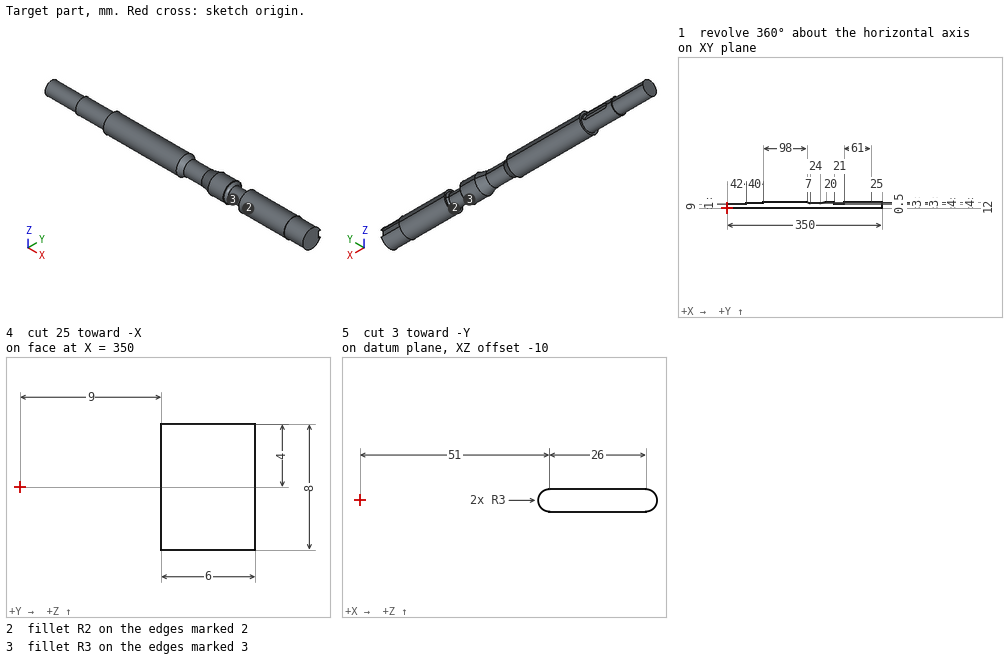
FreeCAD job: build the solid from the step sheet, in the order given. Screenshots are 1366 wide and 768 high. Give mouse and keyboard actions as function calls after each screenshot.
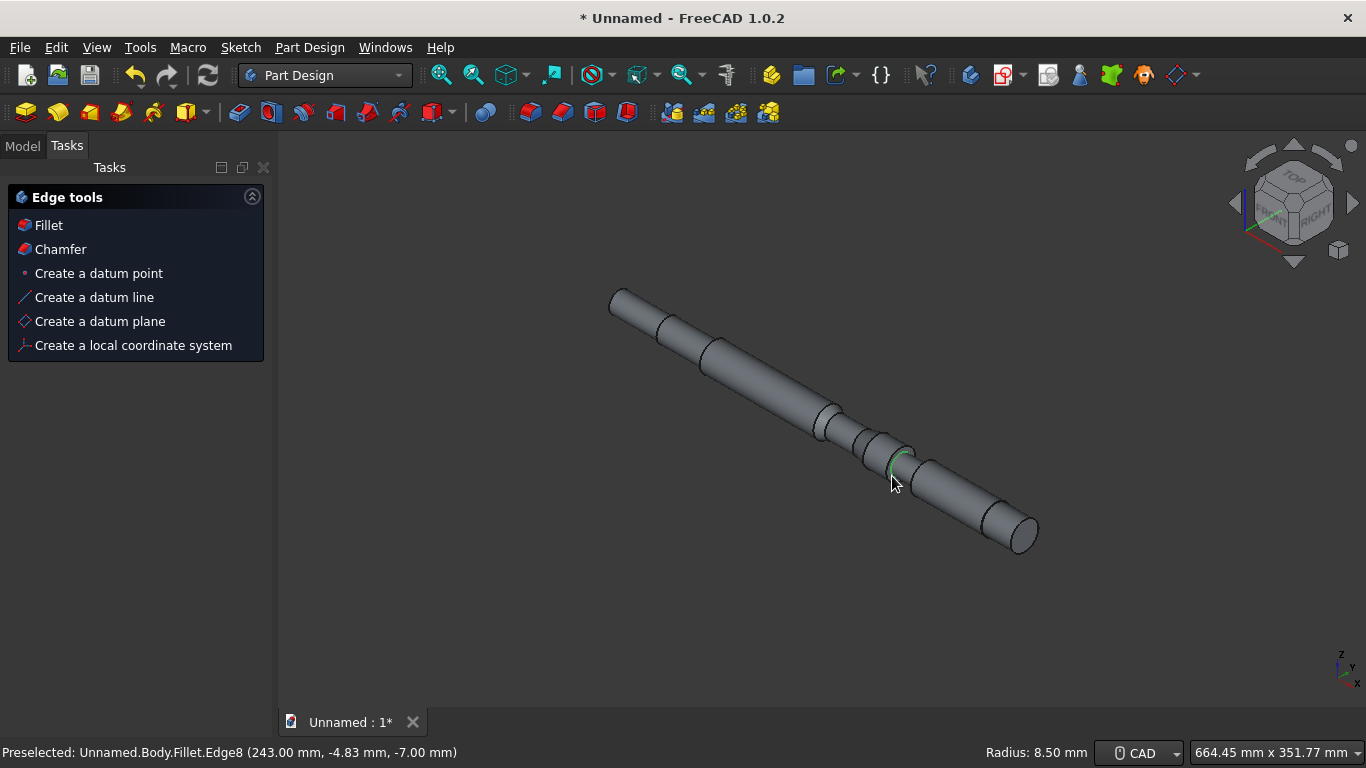
click(532, 112)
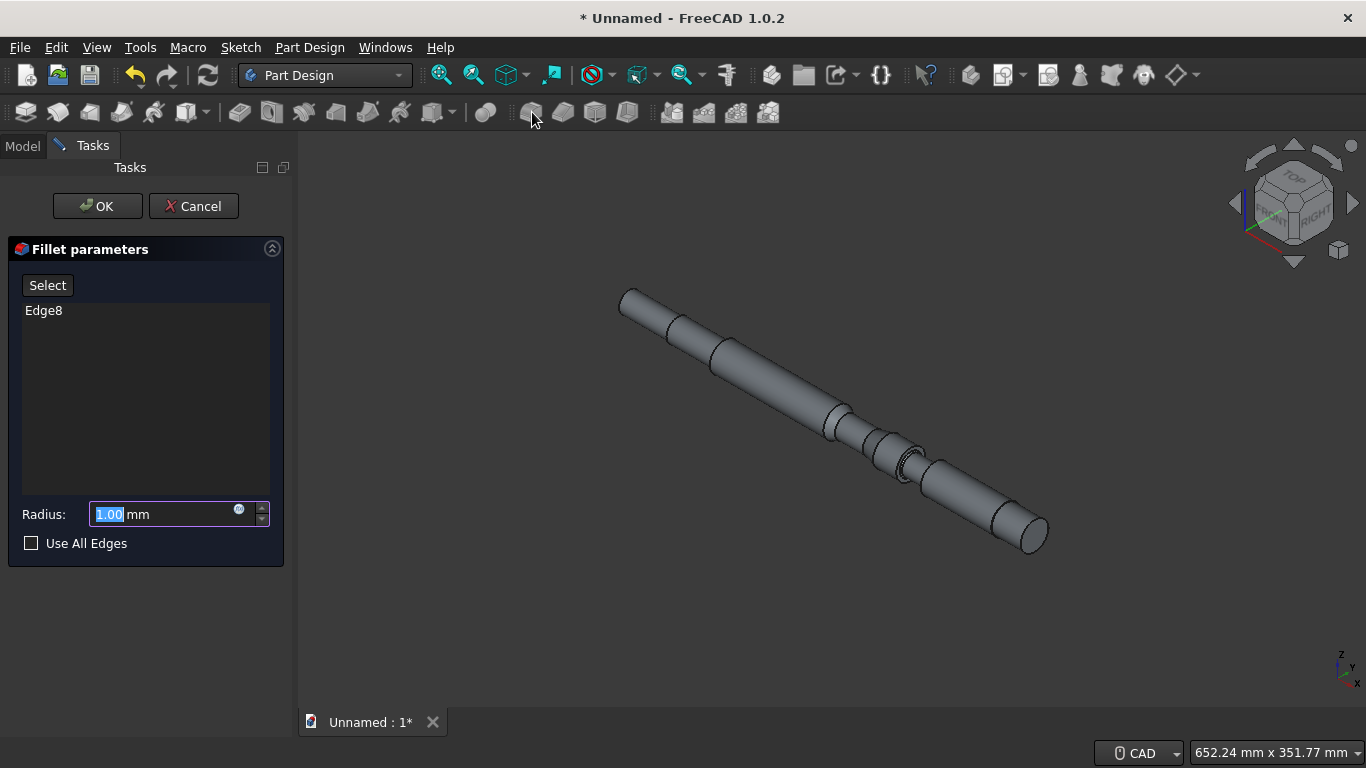
text(3)
key(Tab)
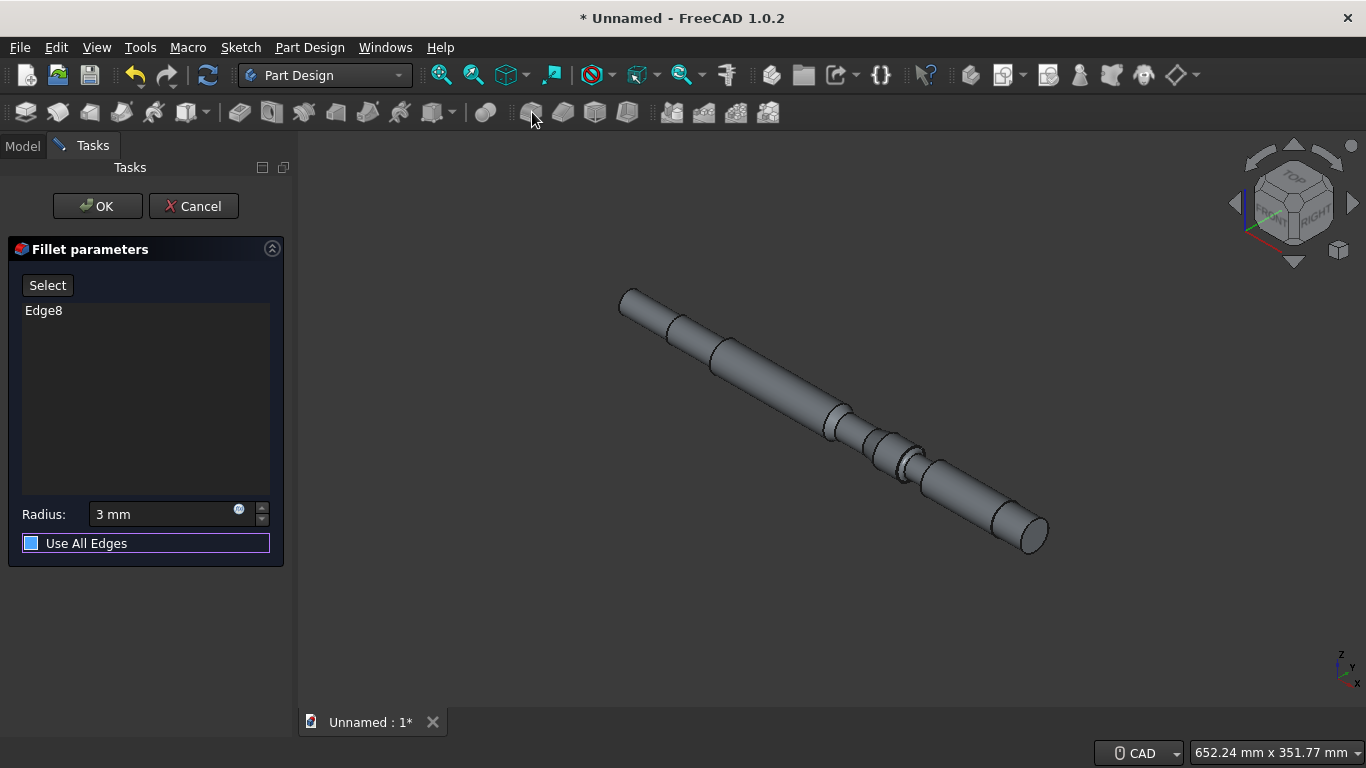
click(98, 206)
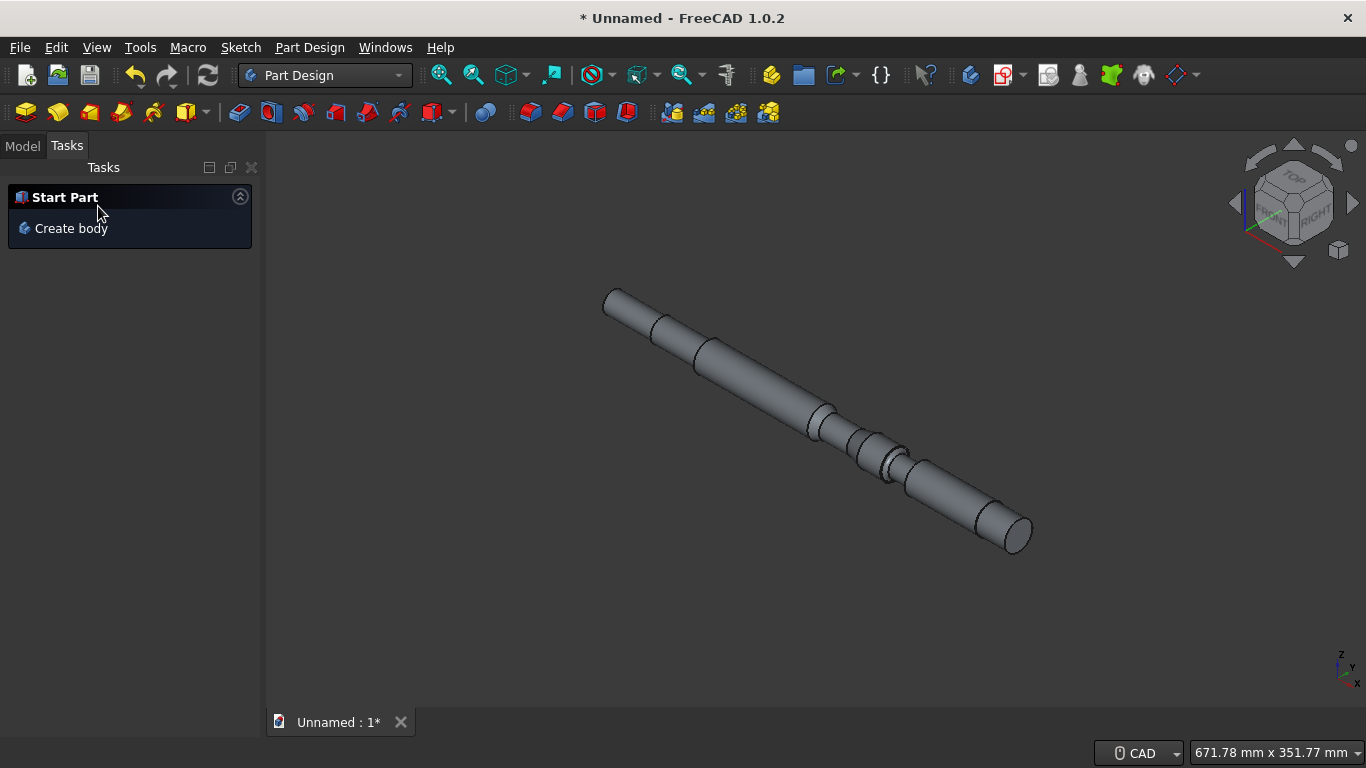
click(1019, 535)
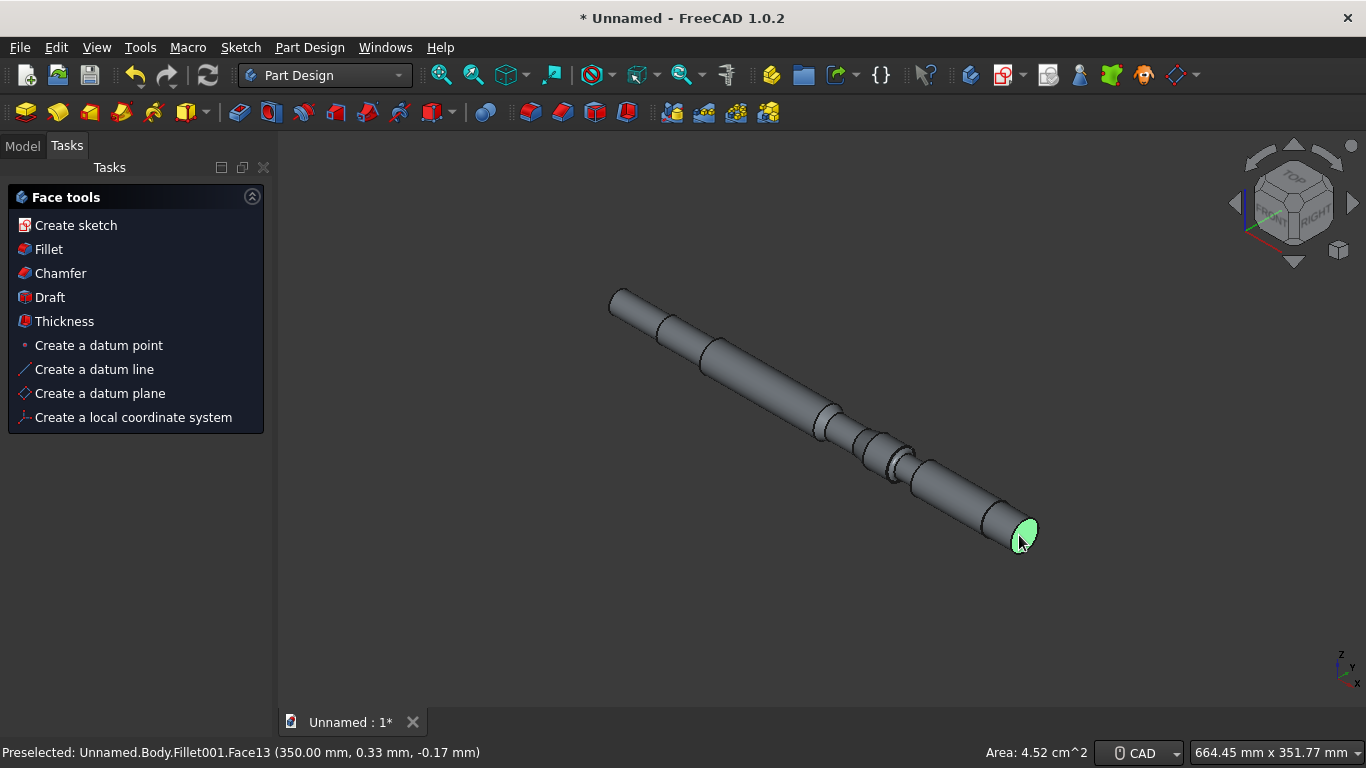
click(1004, 76)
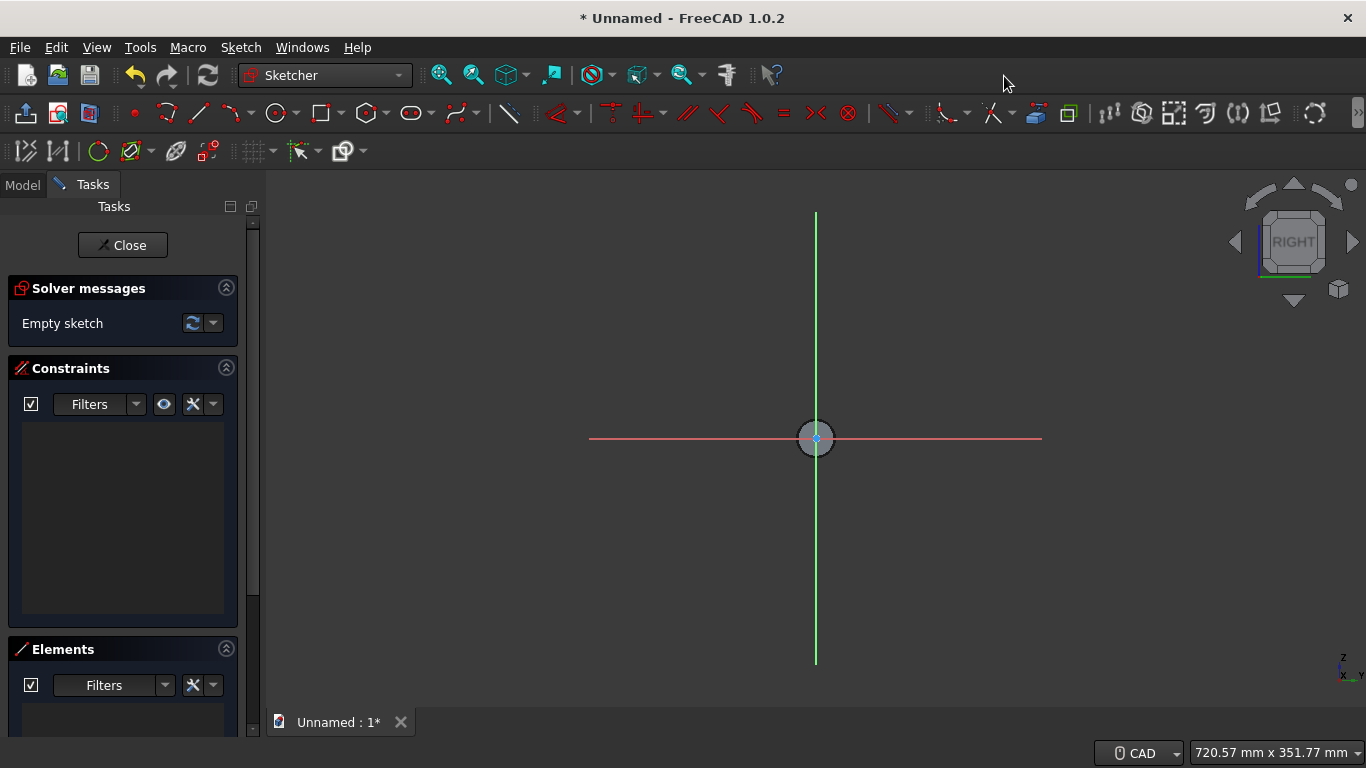
scroll(832, 438, up, 15)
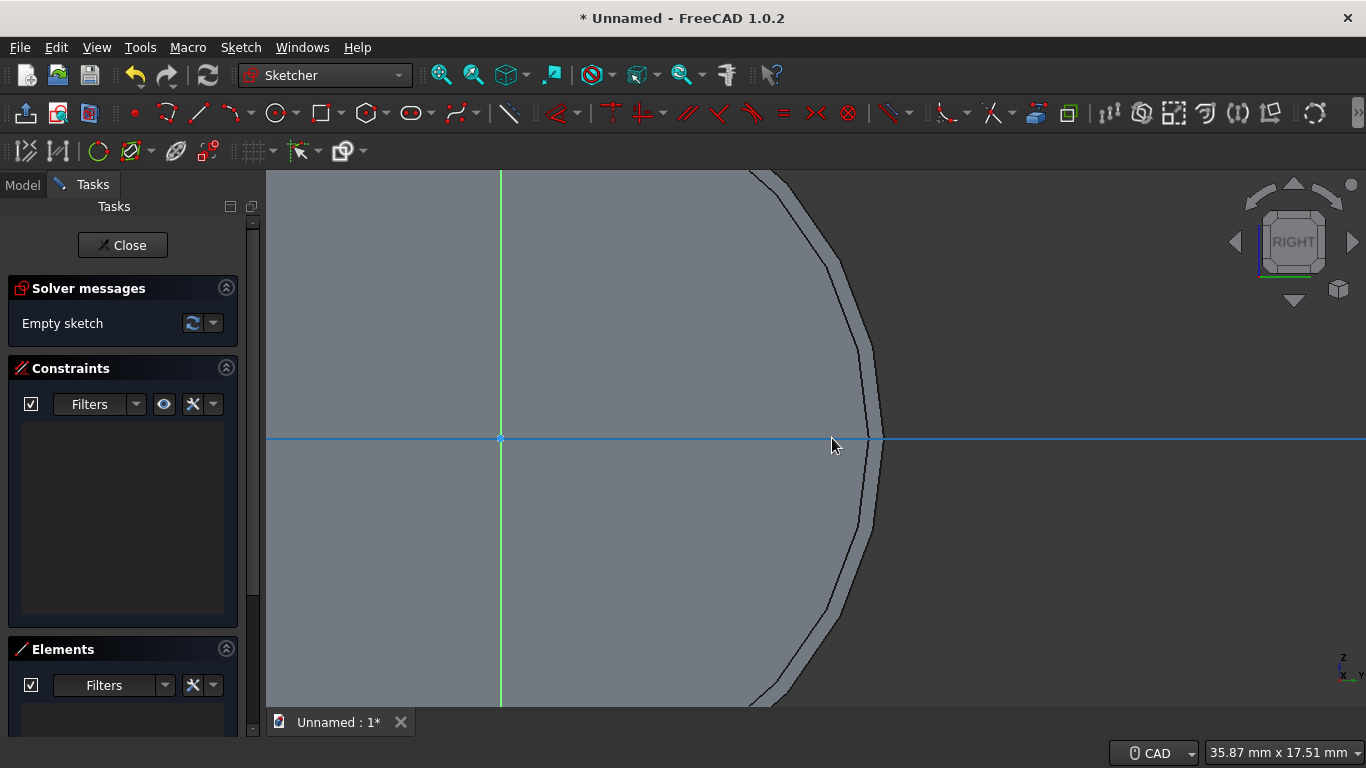
scroll(697, 438, up, 2)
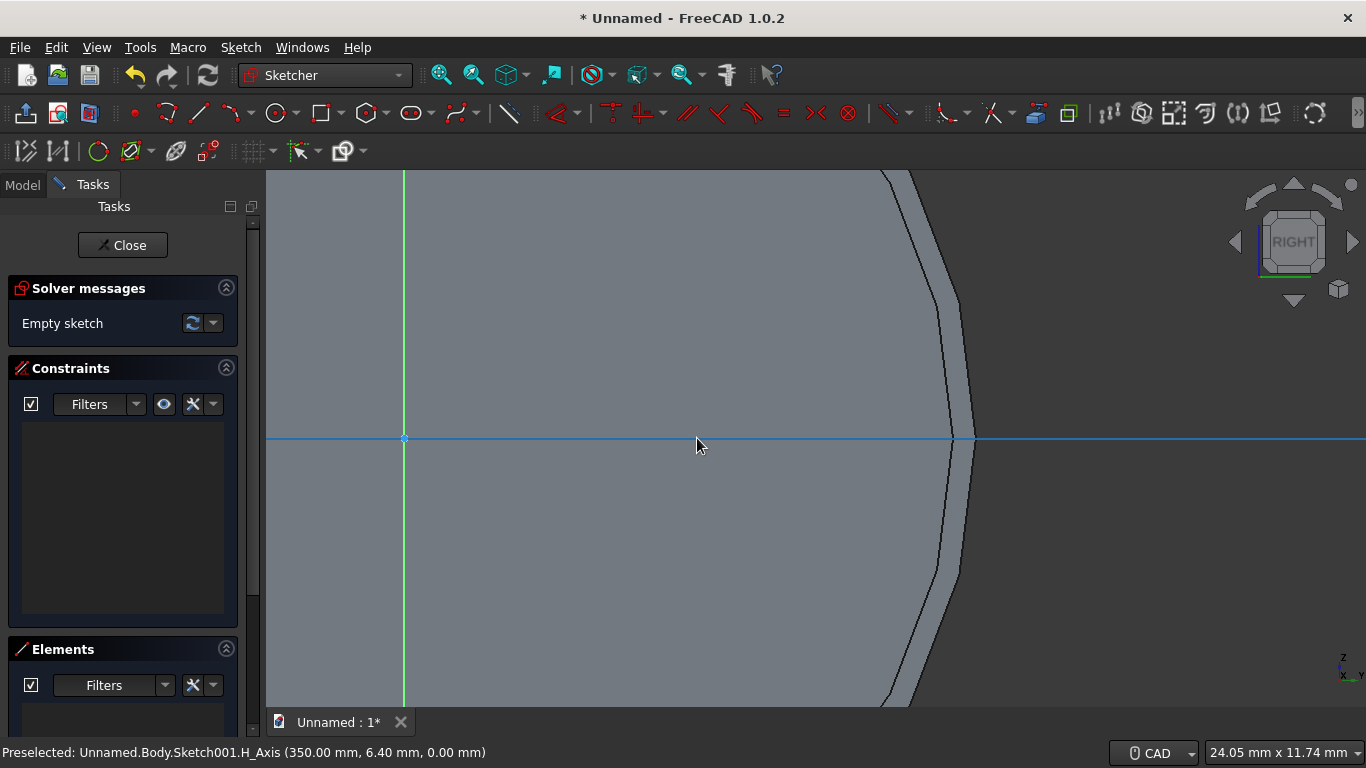
click(322, 114)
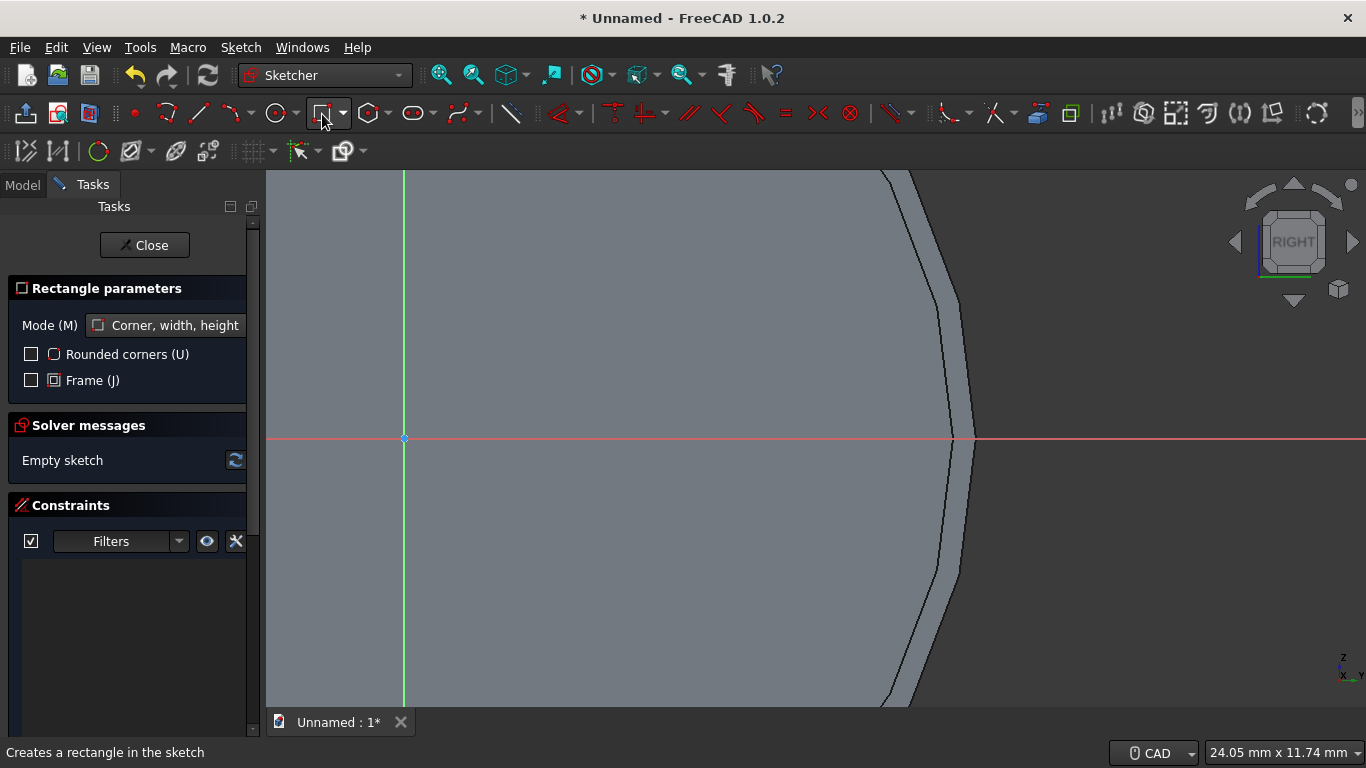
click(816, 256)
move(1090, 621)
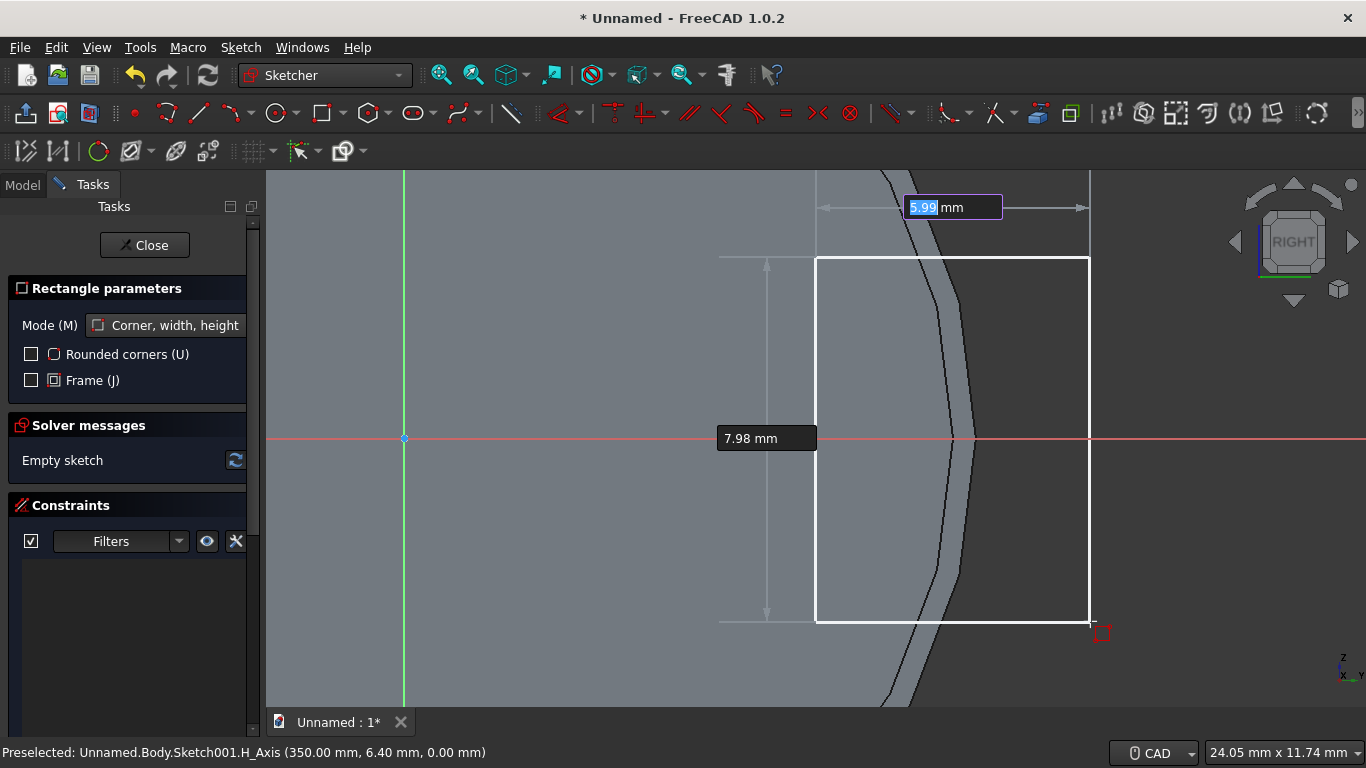
text(6)
key(Tab)
text(8)
key(Return)
key(Escape)